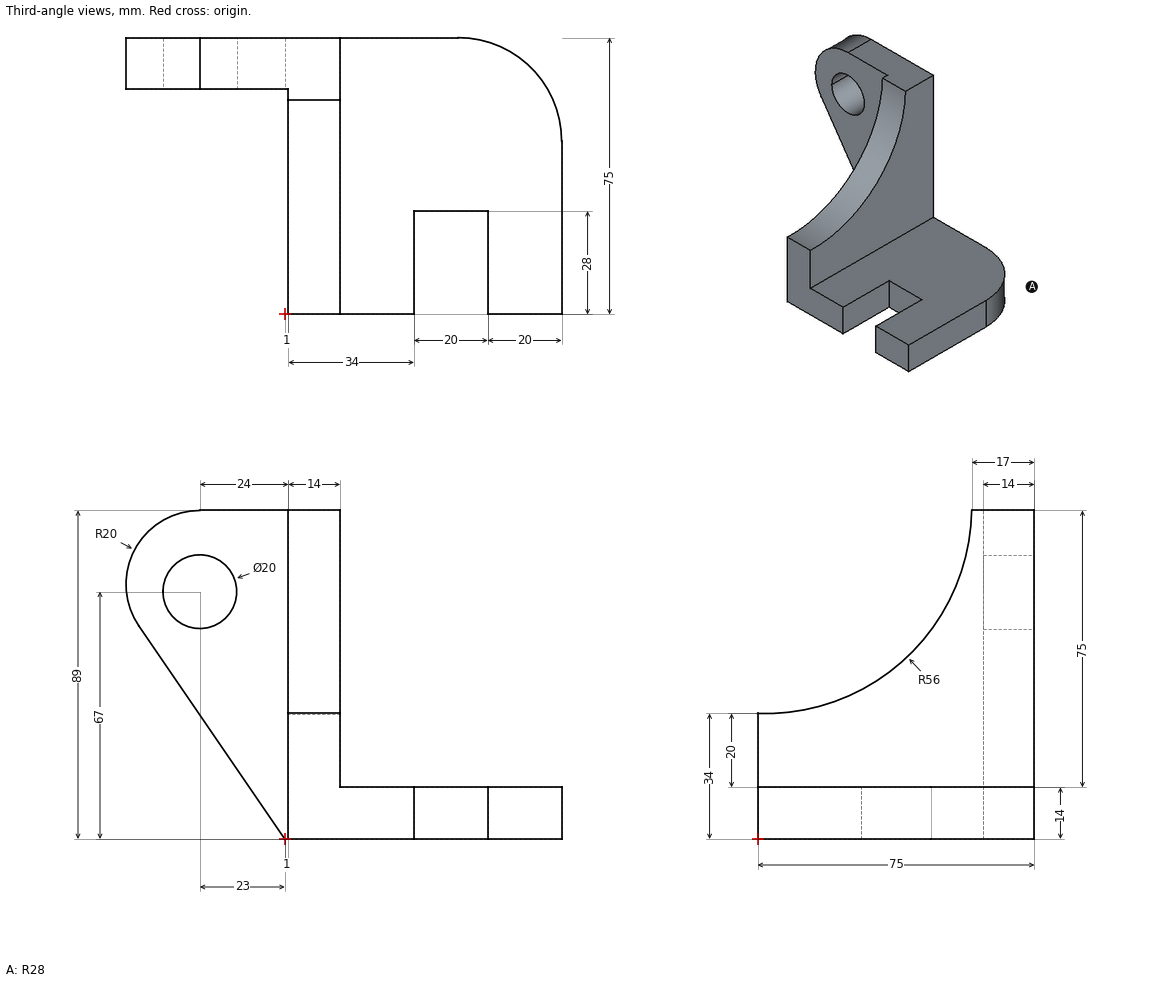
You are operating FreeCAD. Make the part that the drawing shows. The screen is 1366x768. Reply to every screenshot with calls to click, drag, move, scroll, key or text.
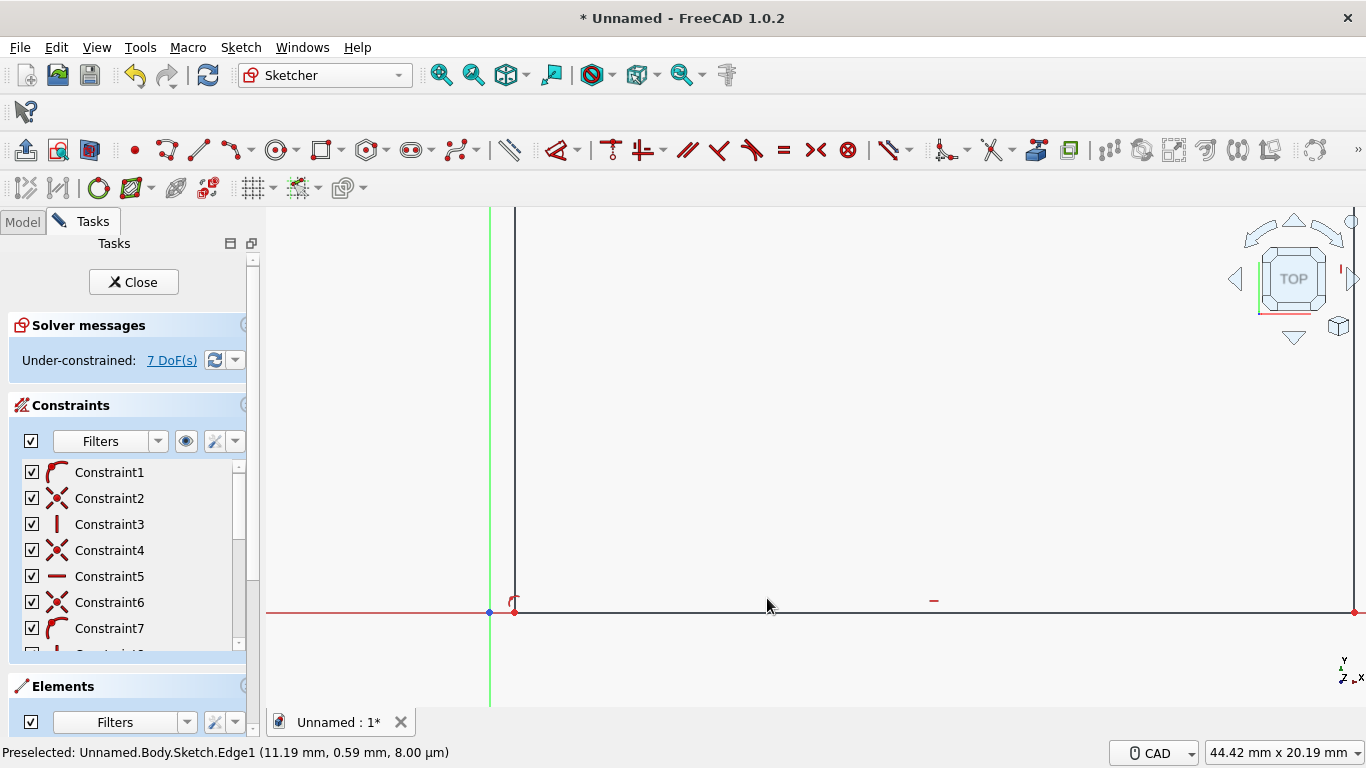
scroll(615, 610, down, 9)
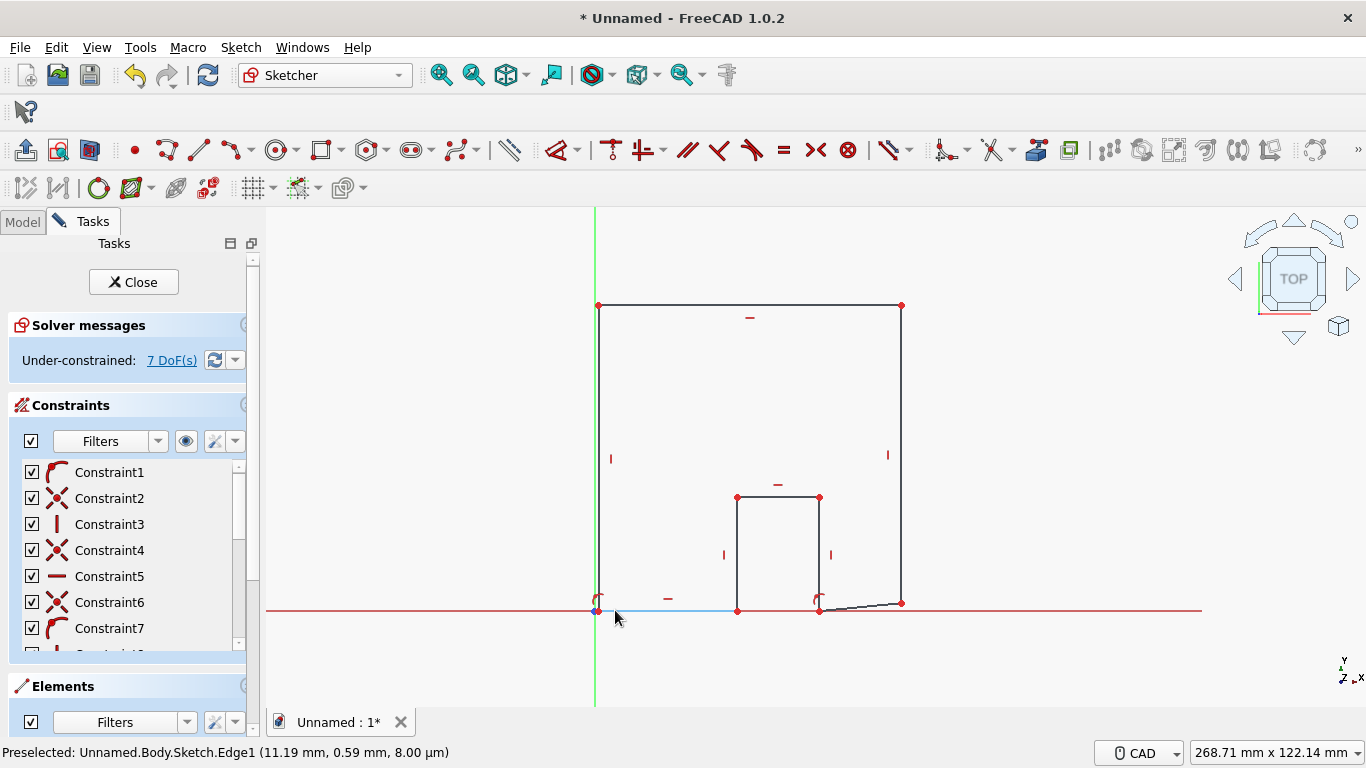
scroll(844, 609, up, 9)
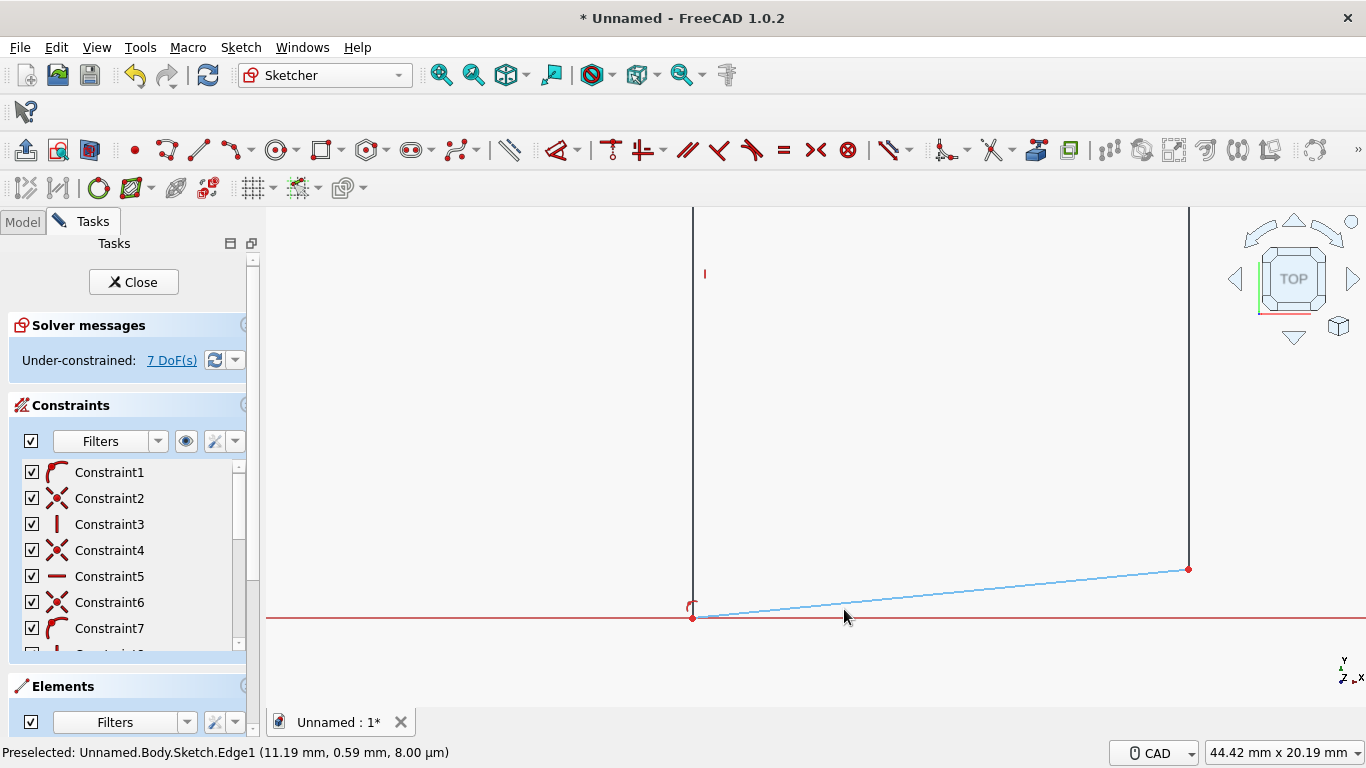
click(842, 603)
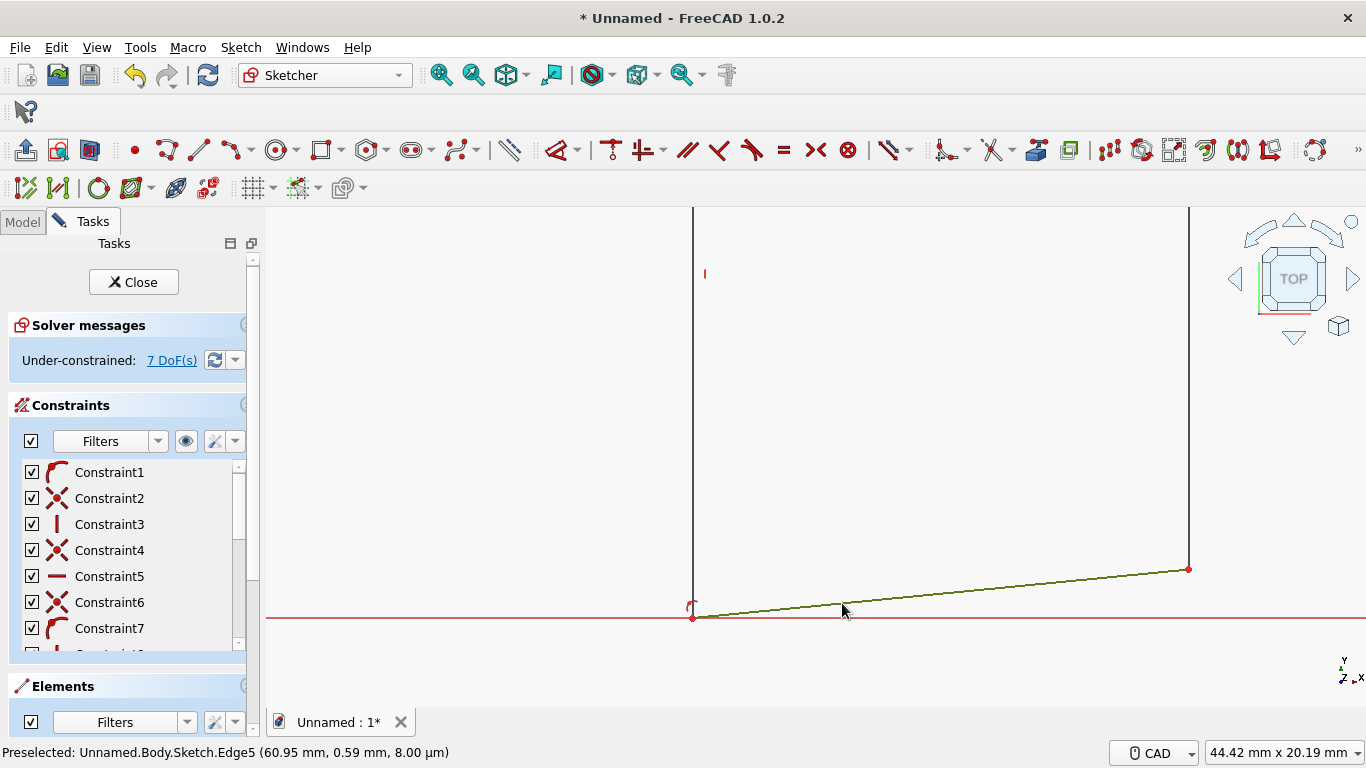
click(666, 150)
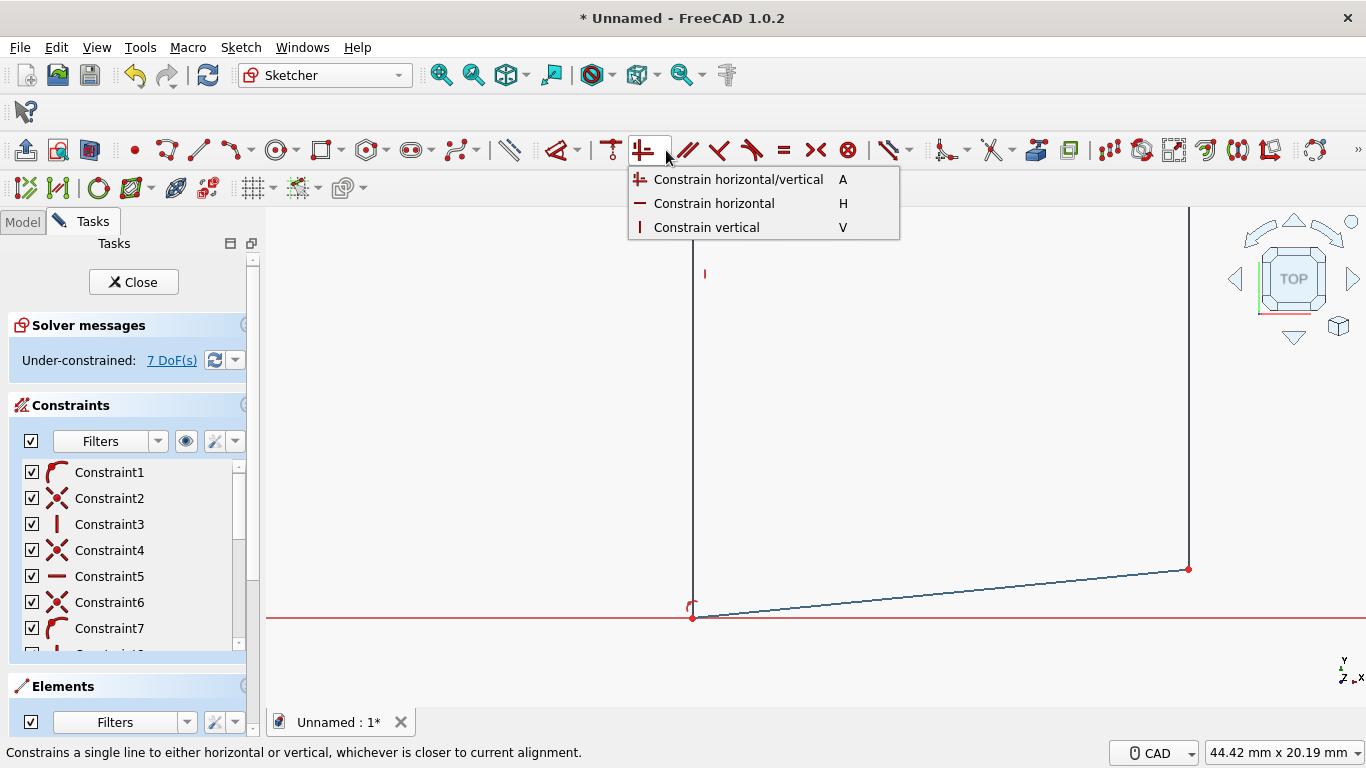
click(764, 203)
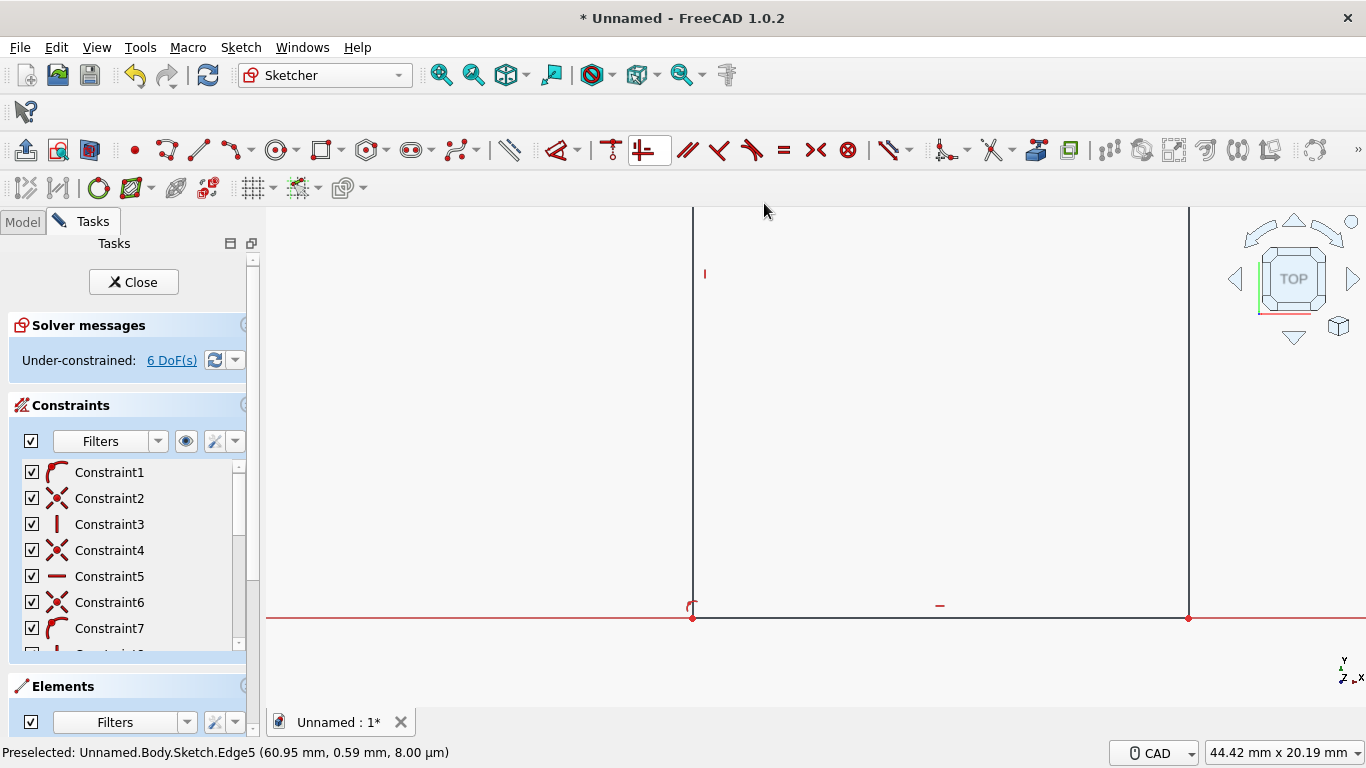
click(556, 150)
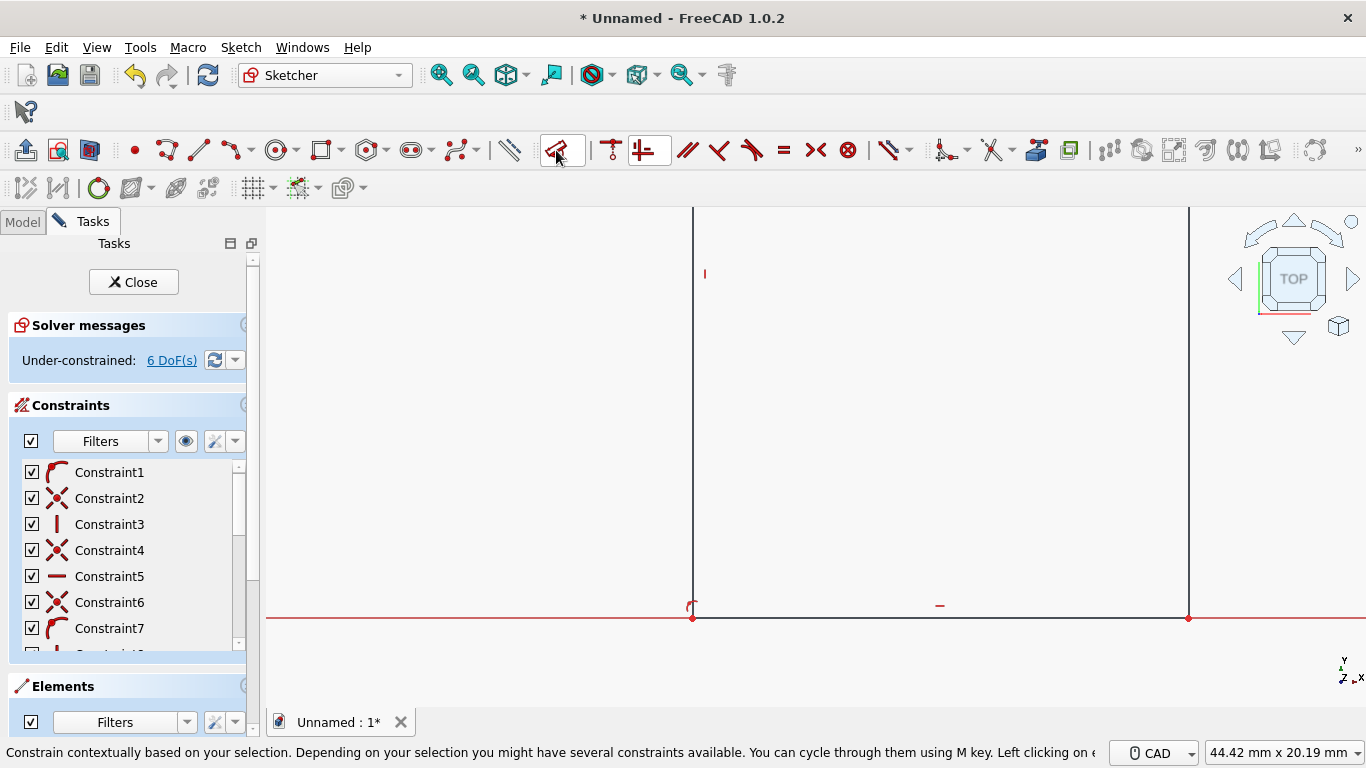
scroll(844, 609, down, 9)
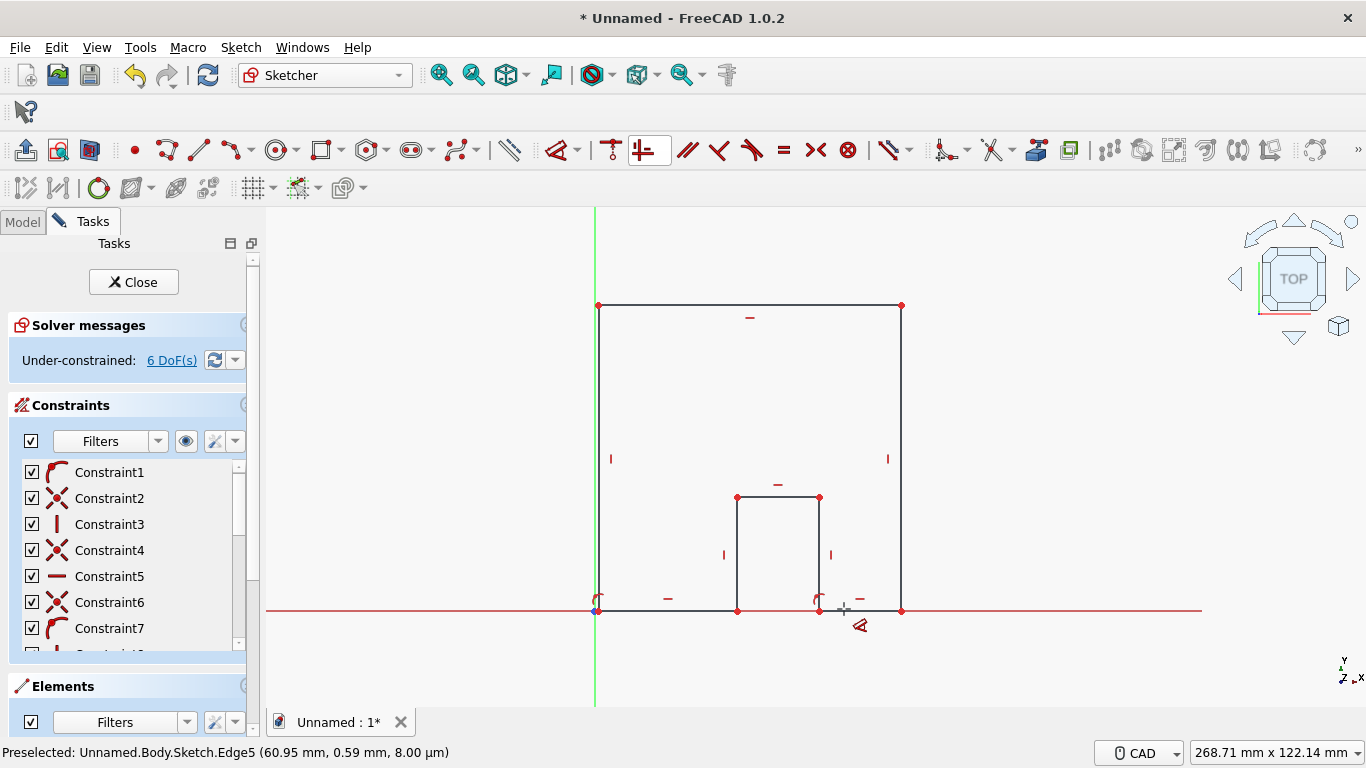
click(640, 611)
click(668, 645)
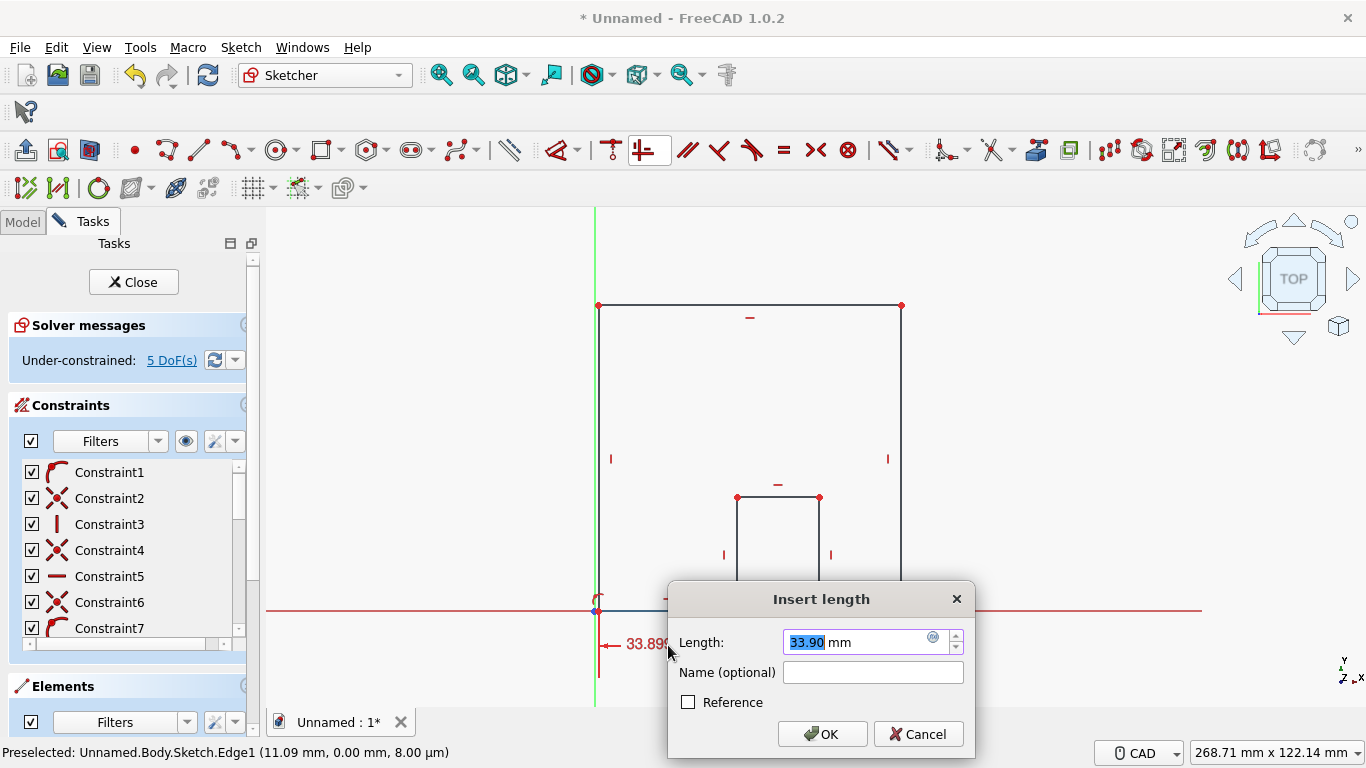
text(34)
key(Return)